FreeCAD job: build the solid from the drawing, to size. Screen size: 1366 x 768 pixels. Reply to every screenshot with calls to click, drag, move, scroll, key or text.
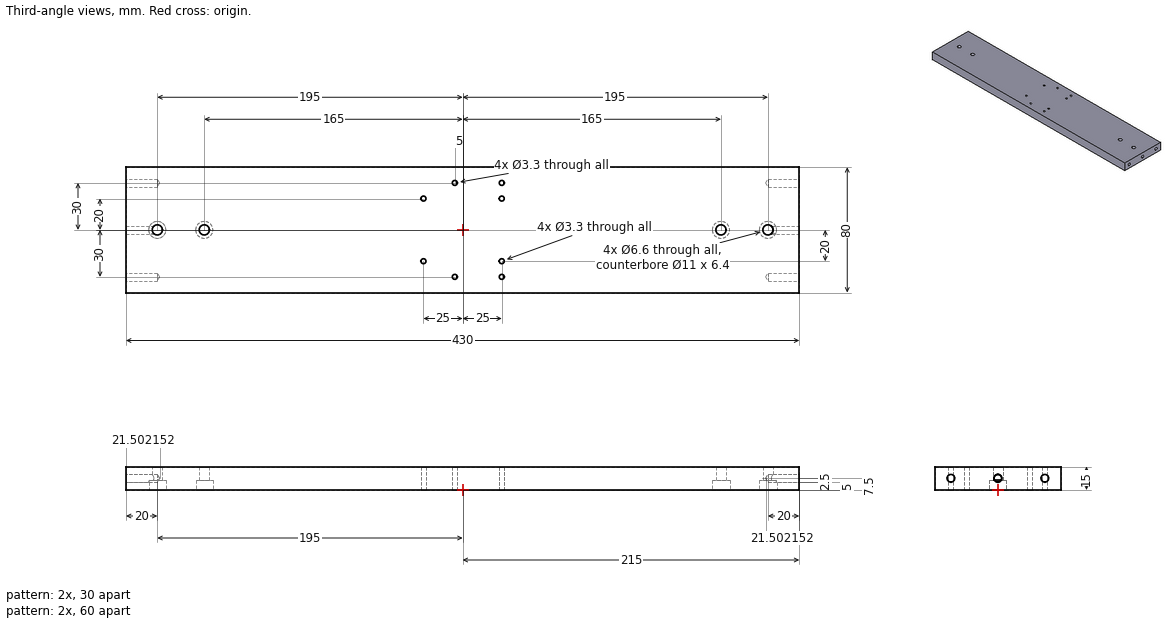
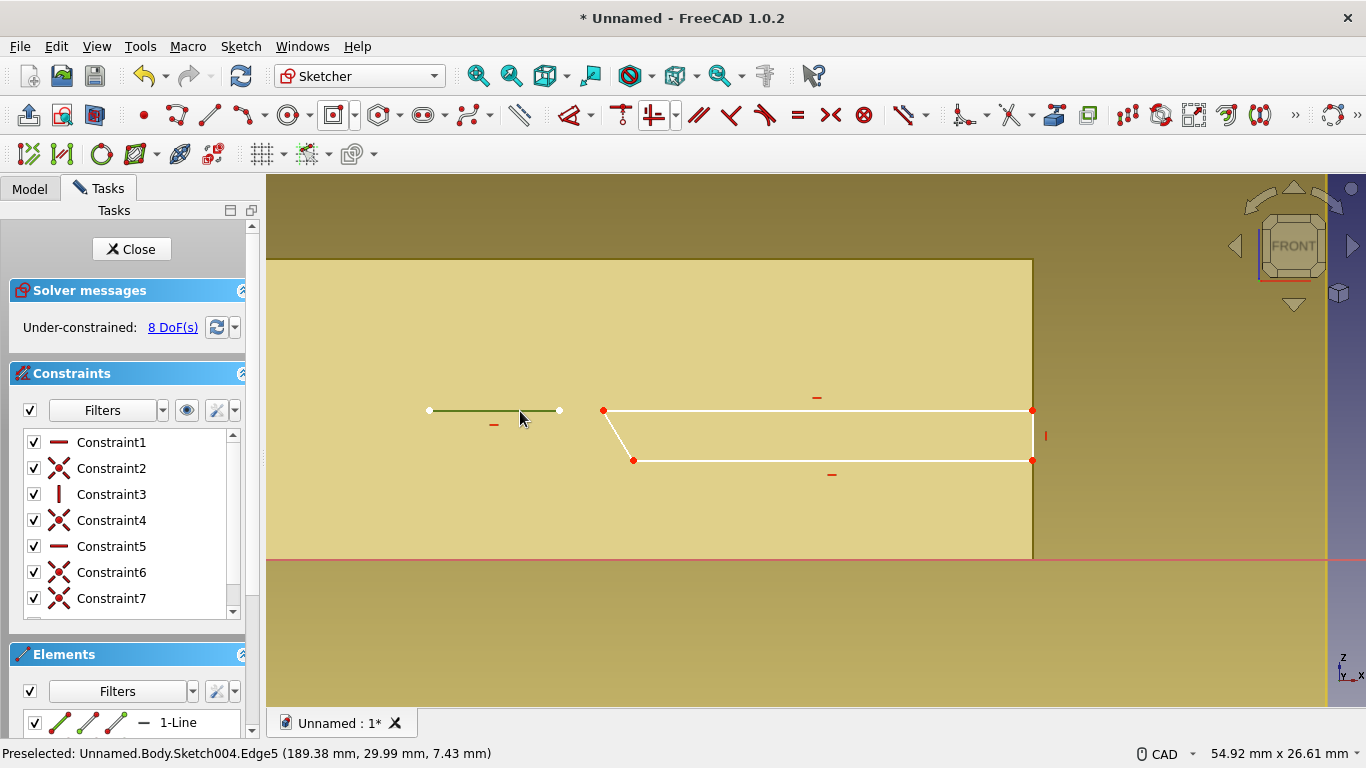
click(520, 116)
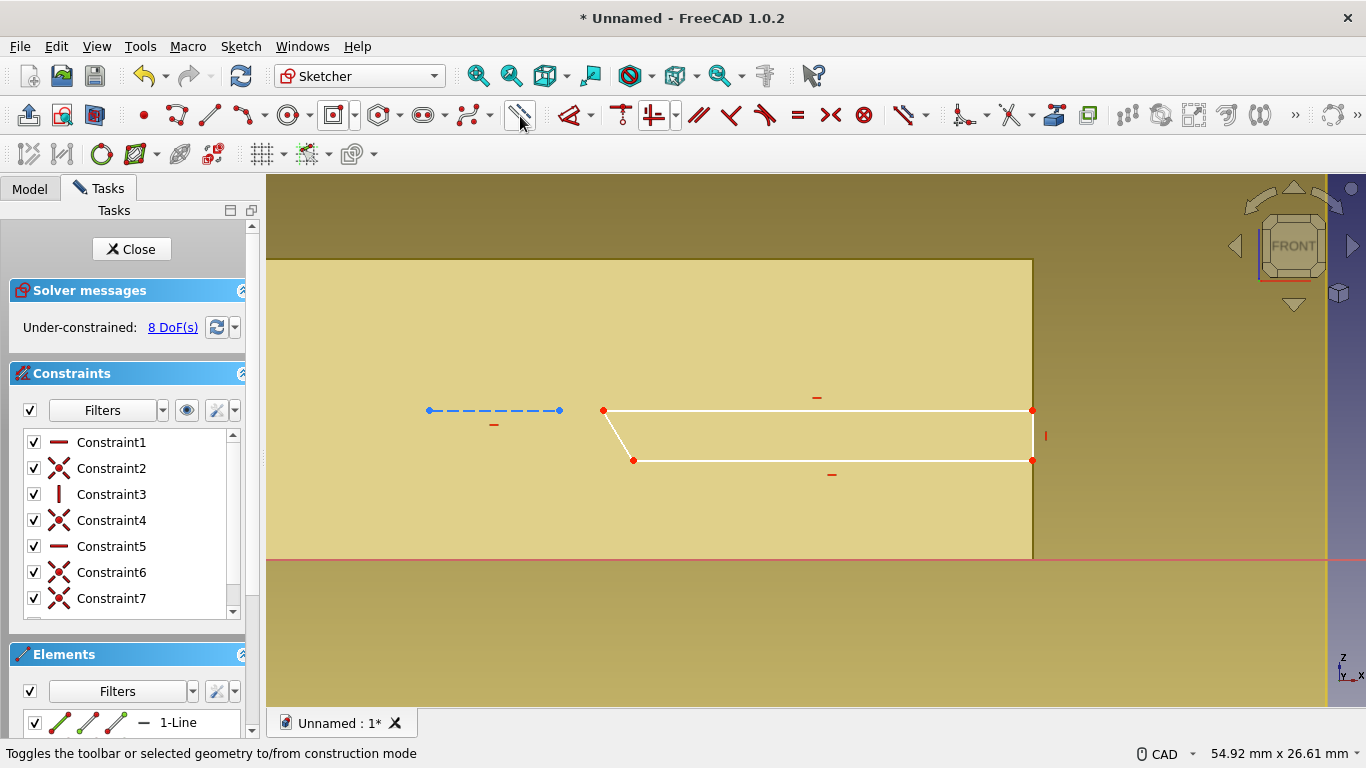
key(d)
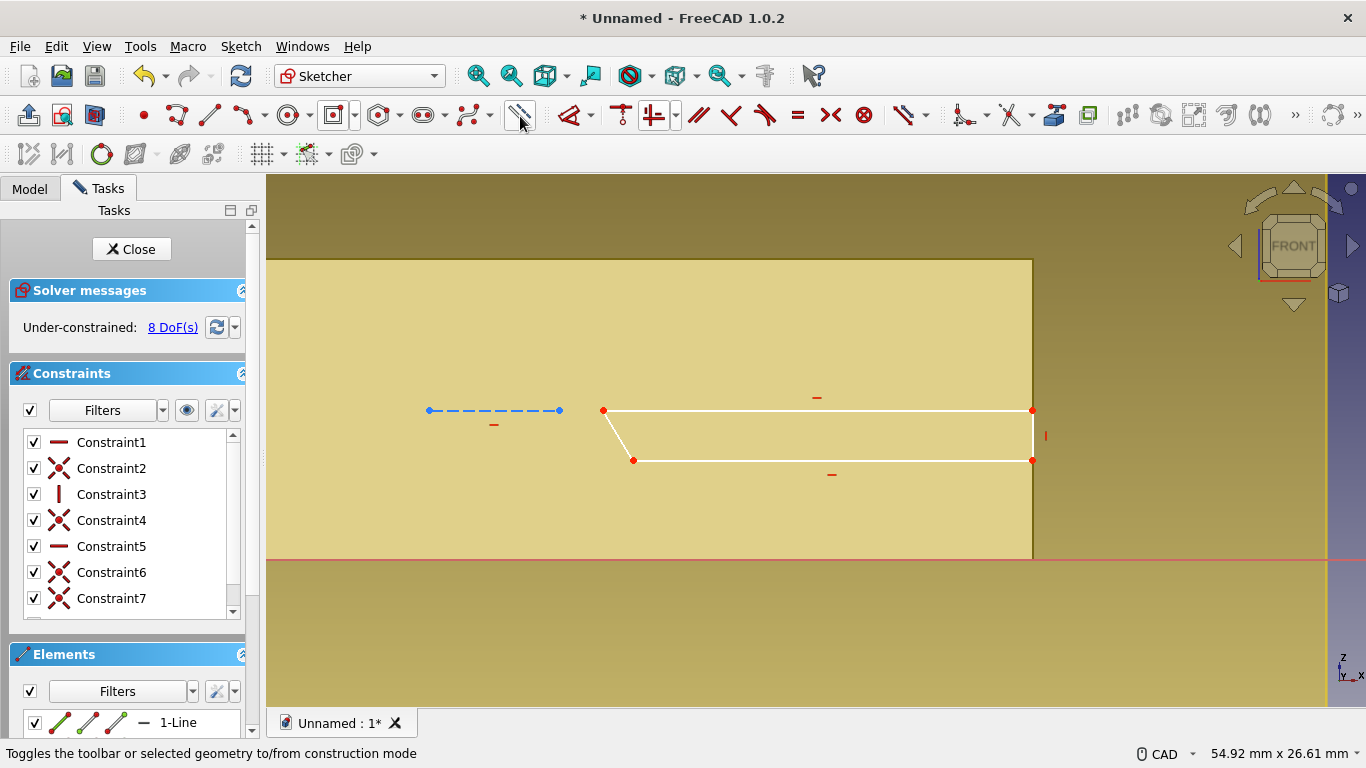
click(913, 461)
click(833, 495)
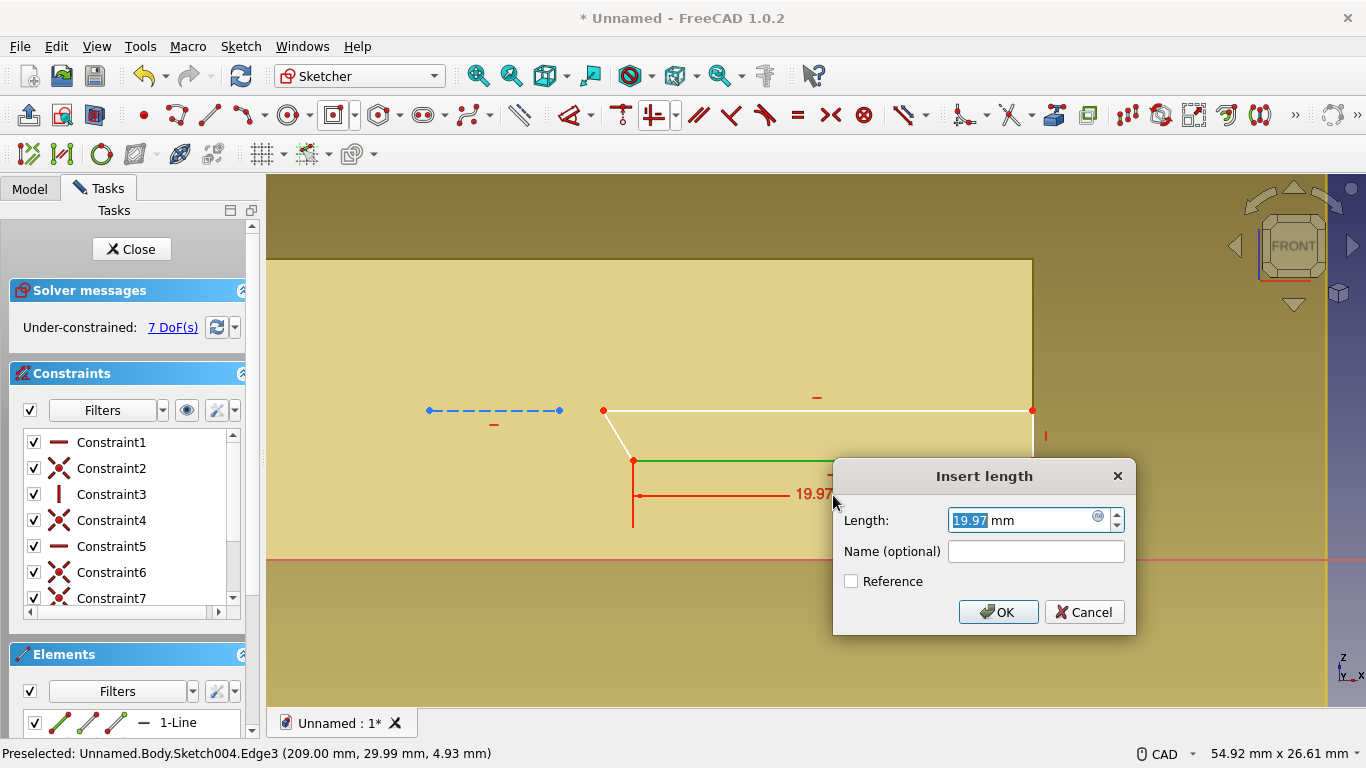
text(20)
key(Return)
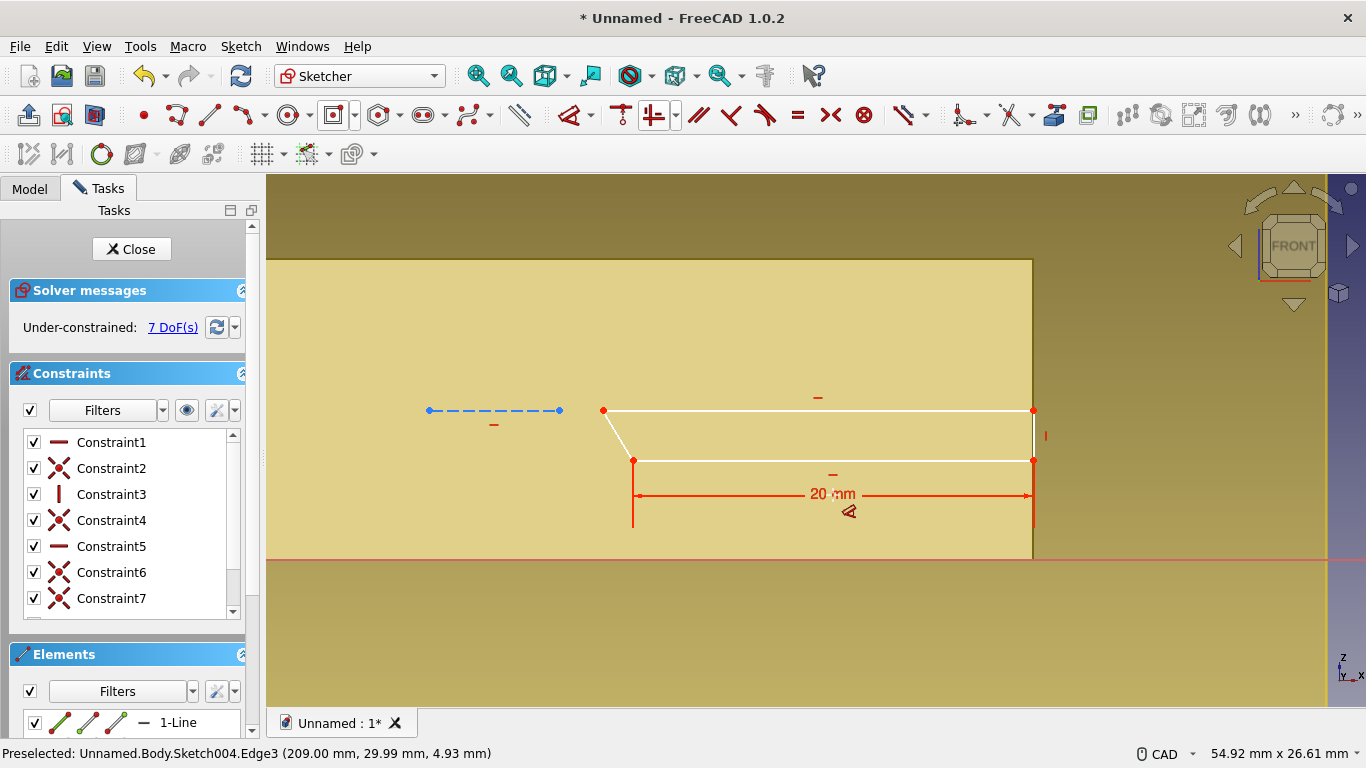
click(1034, 461)
click(1068, 510)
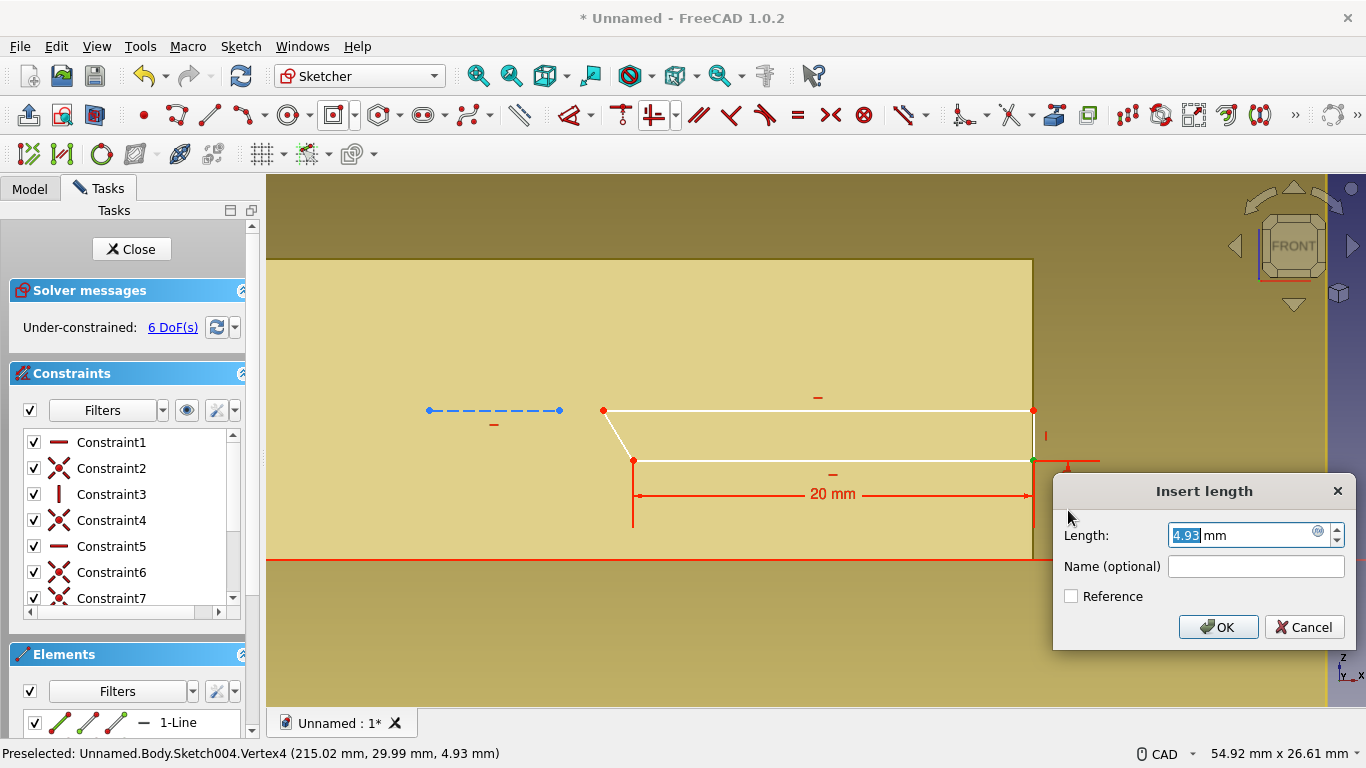
text(5)
key(Return)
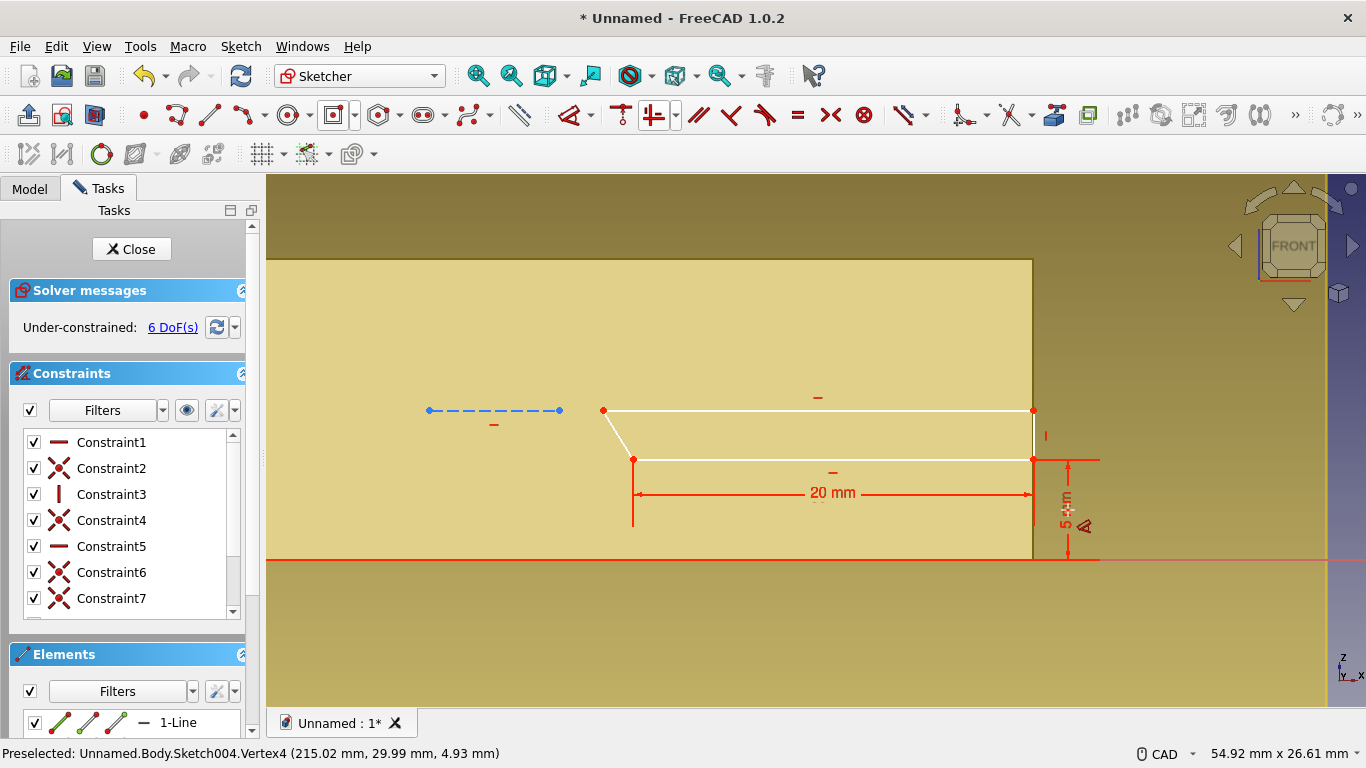
click(1034, 426)
click(1068, 435)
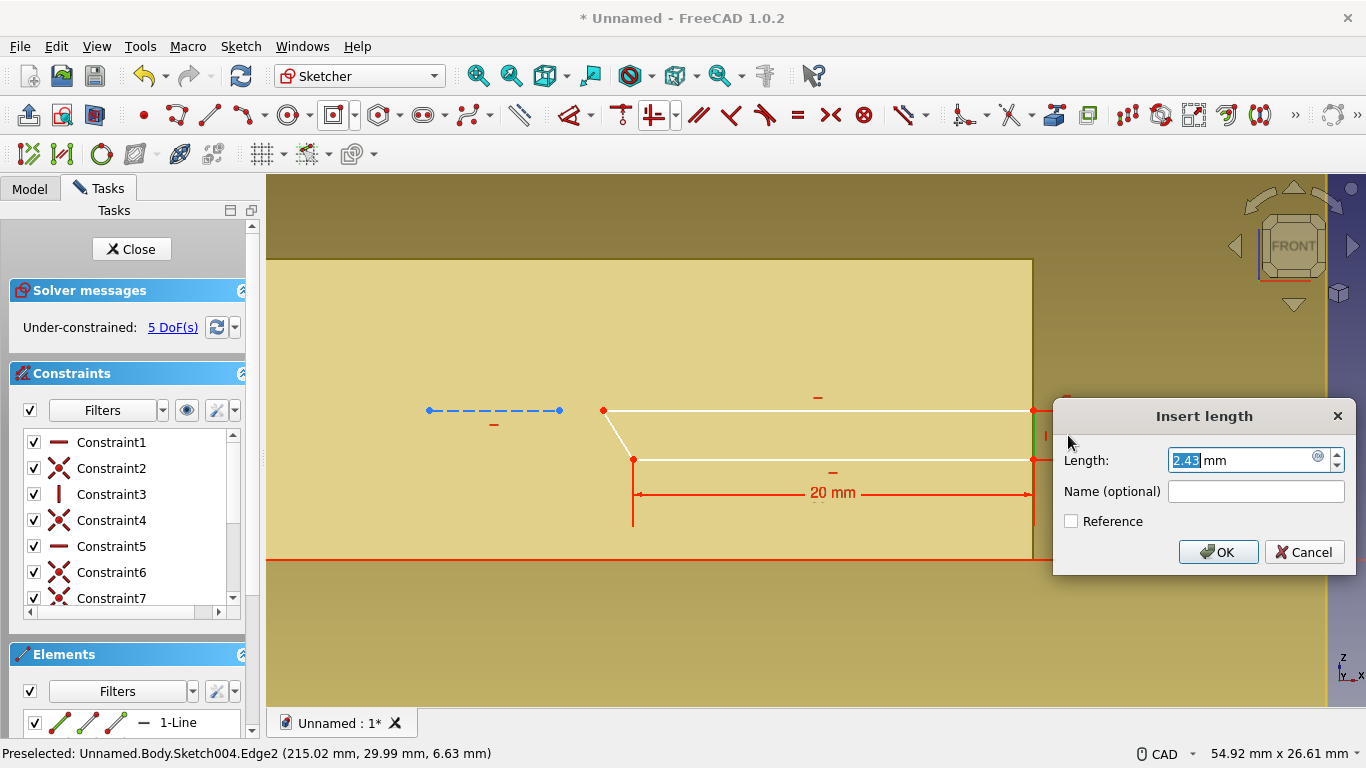
text(2.5)
key(Return)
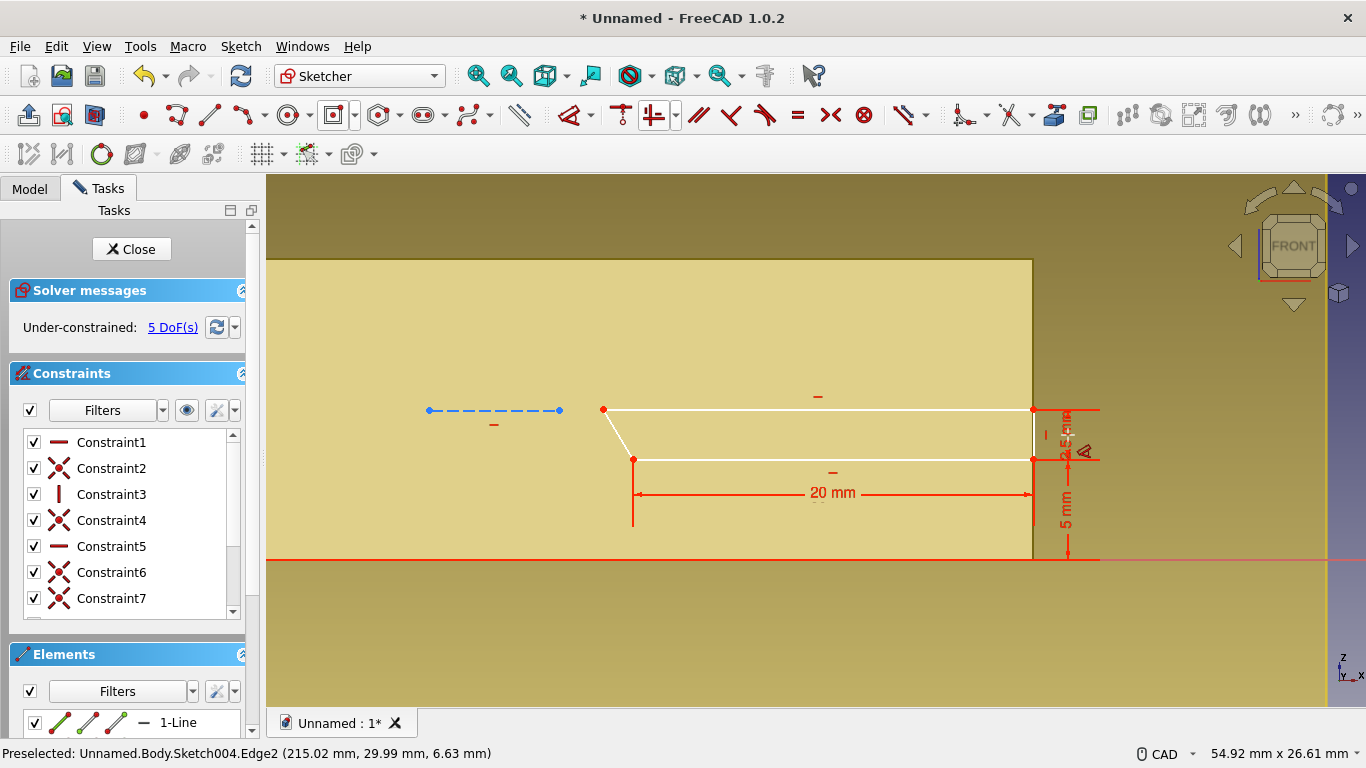
click(1034, 410)
click(664, 594)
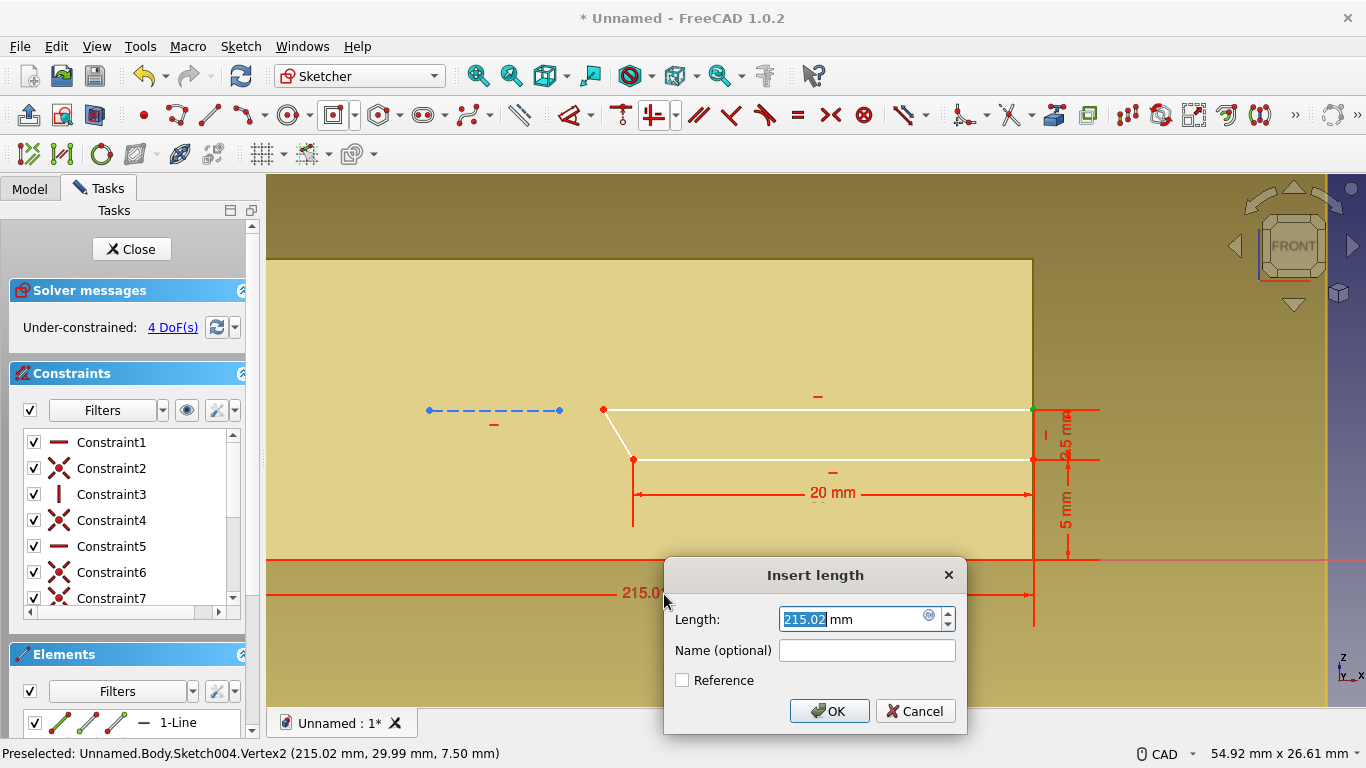
text(215)
key(Return)